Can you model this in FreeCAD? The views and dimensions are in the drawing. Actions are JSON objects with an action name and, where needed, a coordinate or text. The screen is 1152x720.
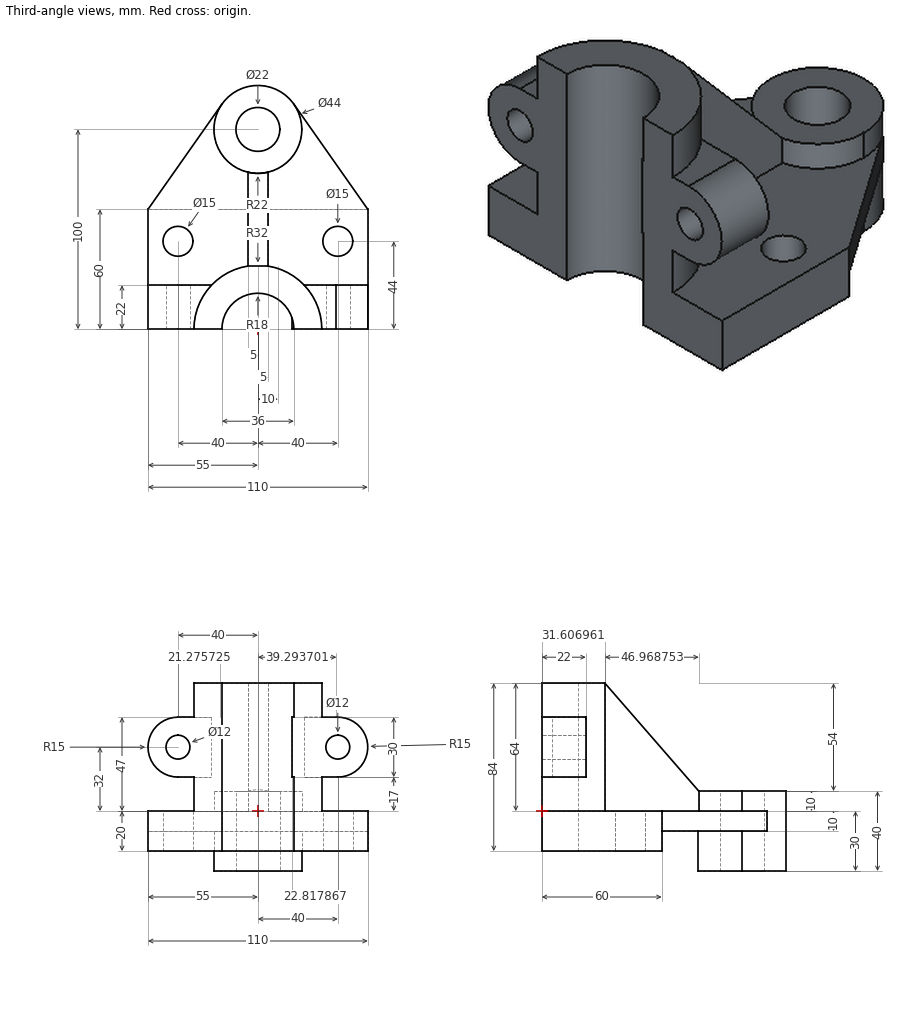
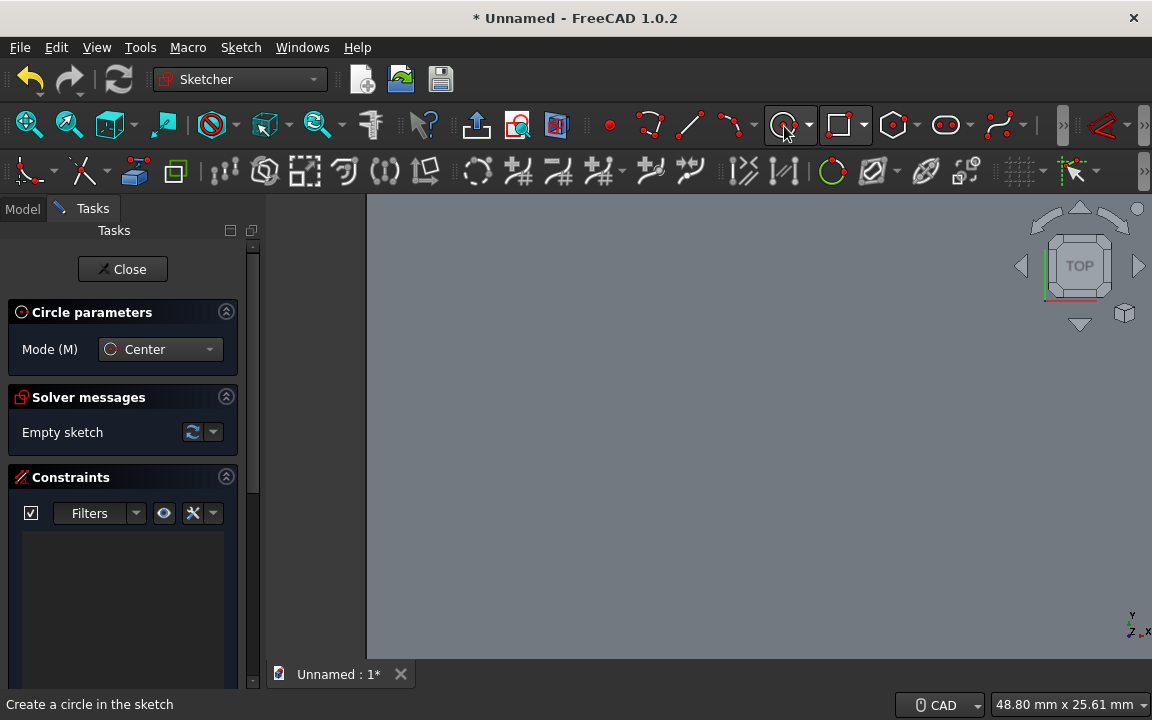
{"action": "left_click", "coordinate": [638, 421]}
{"action": "left_click", "coordinate": [735, 325]}
{"action": "key", "text": "Escape"}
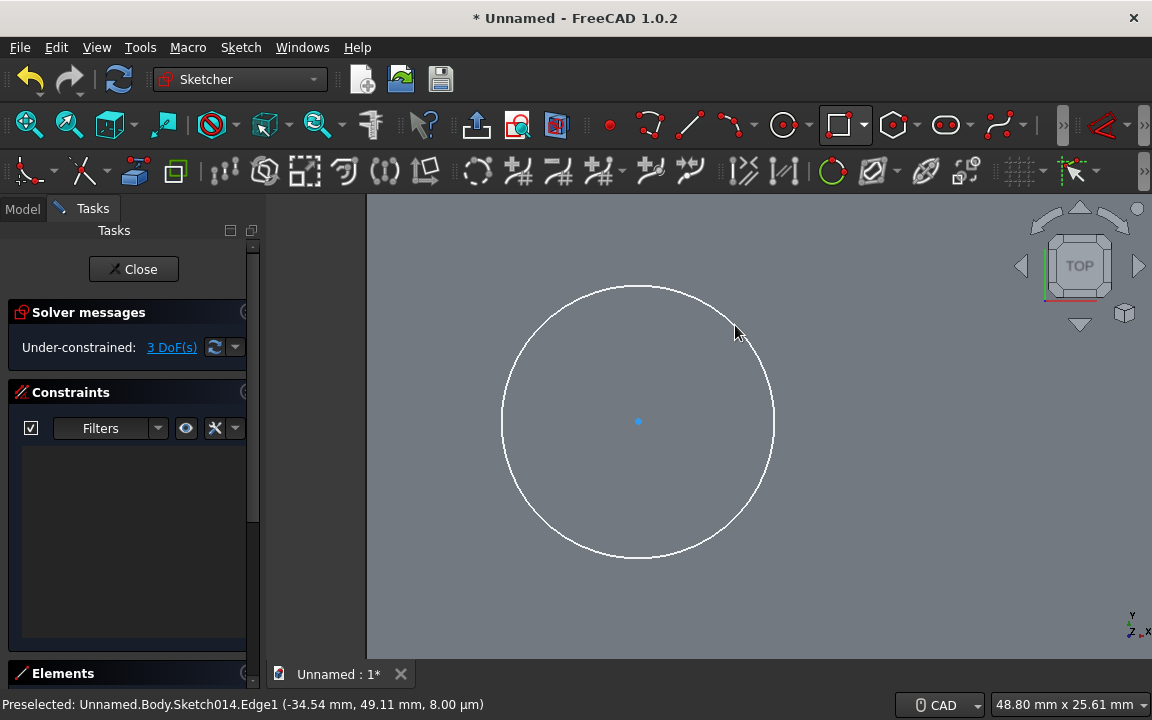
{"action": "left_click", "coordinate": [1102, 126]}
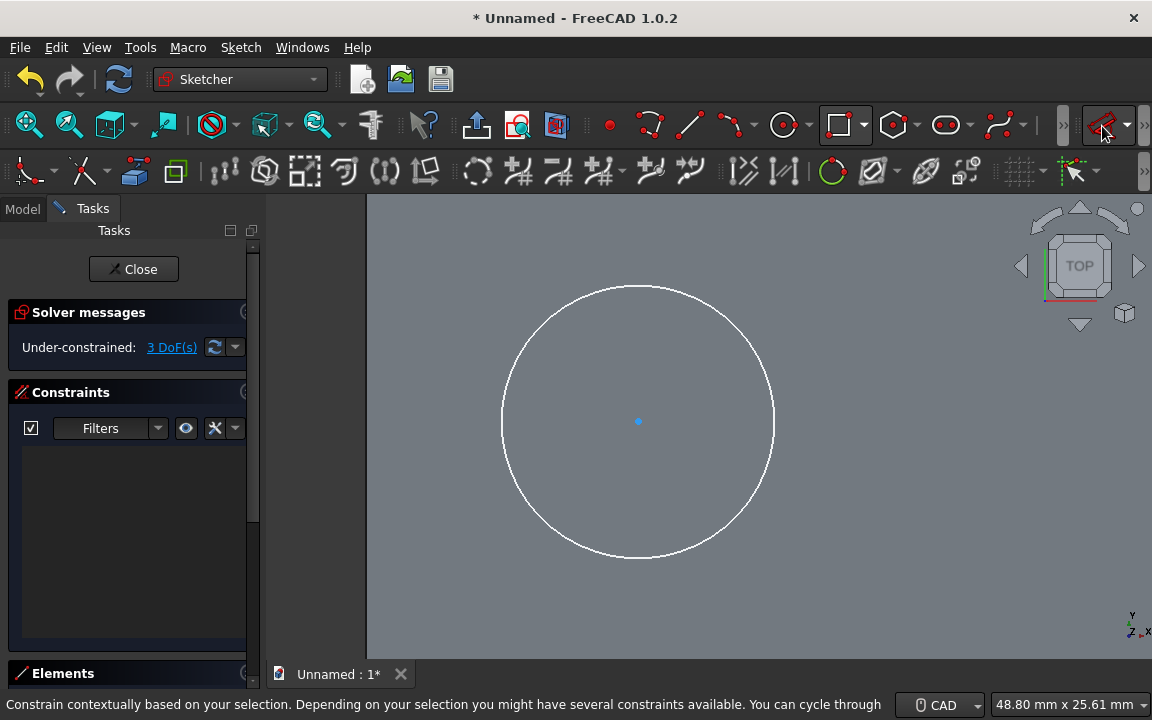
{"action": "left_click", "coordinate": [734, 325]}
{"action": "left_click", "coordinate": [757, 302]}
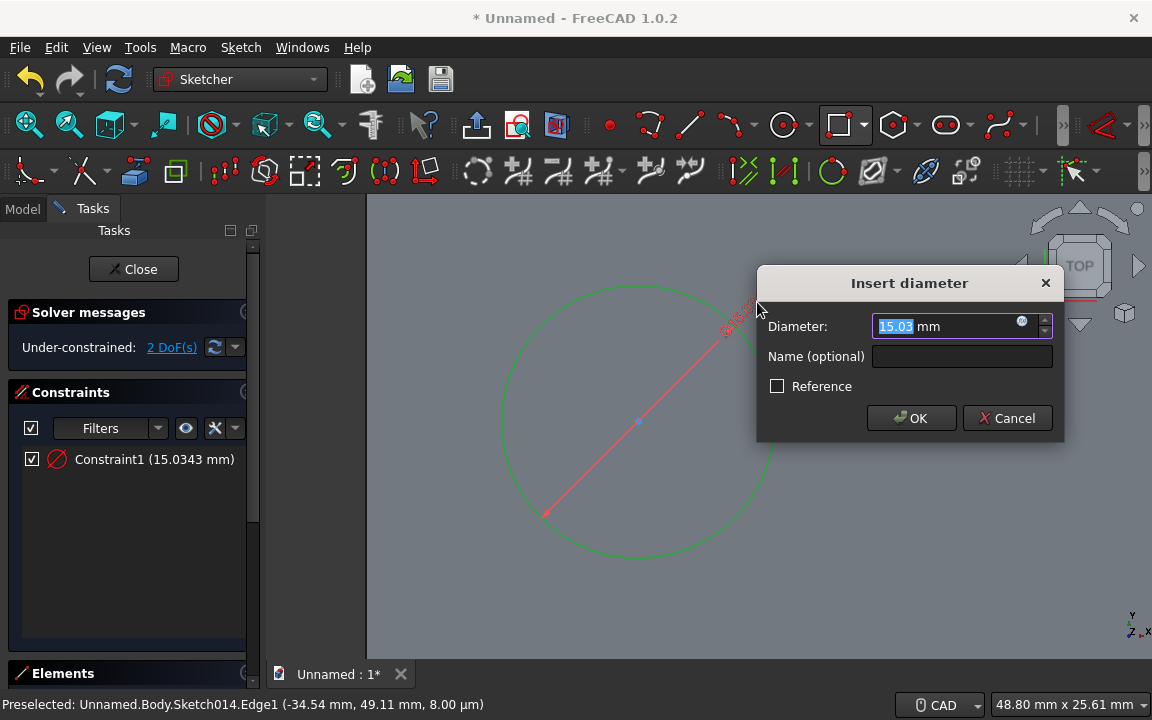
{"action": "type", "text": "15"}
{"action": "key", "text": "Return"}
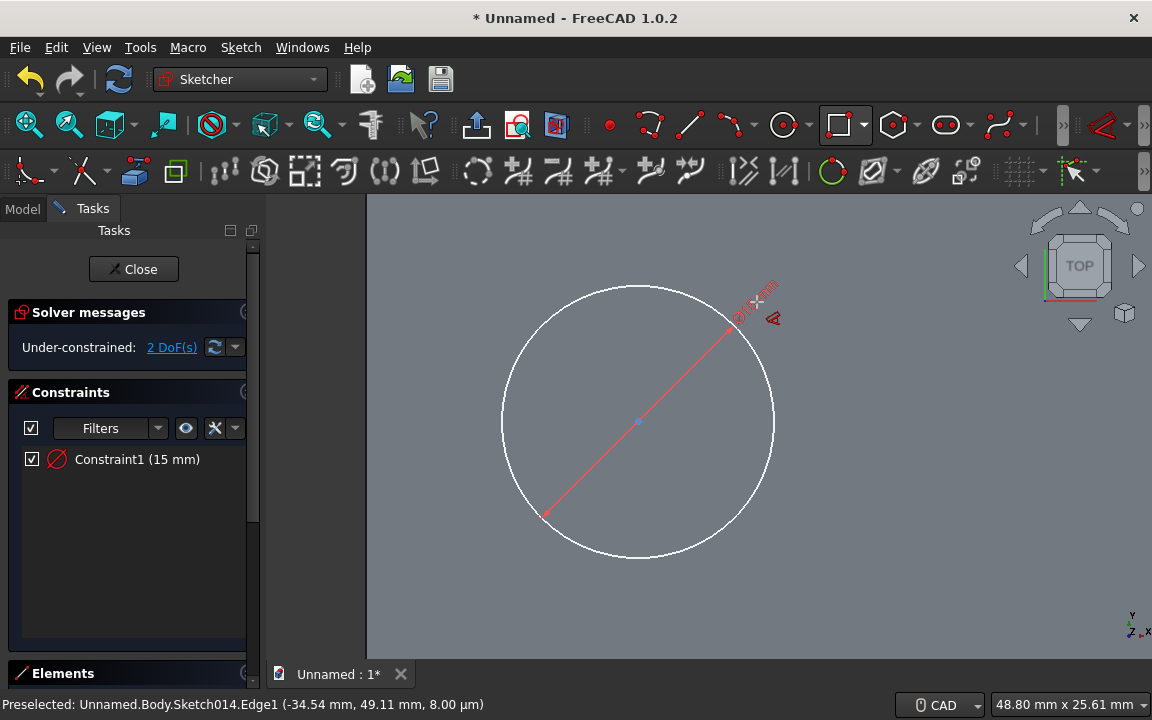
{"action": "left_click", "coordinate": [638, 422]}
{"action": "left_click", "coordinate": [812, 388]}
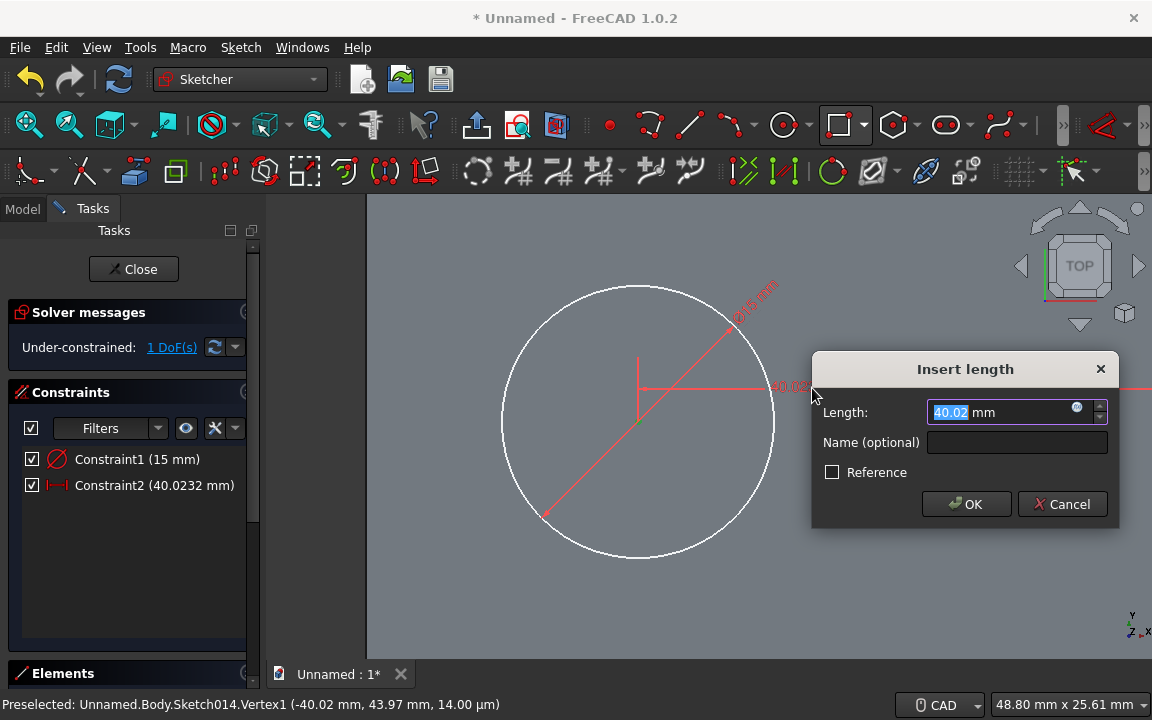
{"action": "type", "text": "40"}
{"action": "key", "text": "Return"}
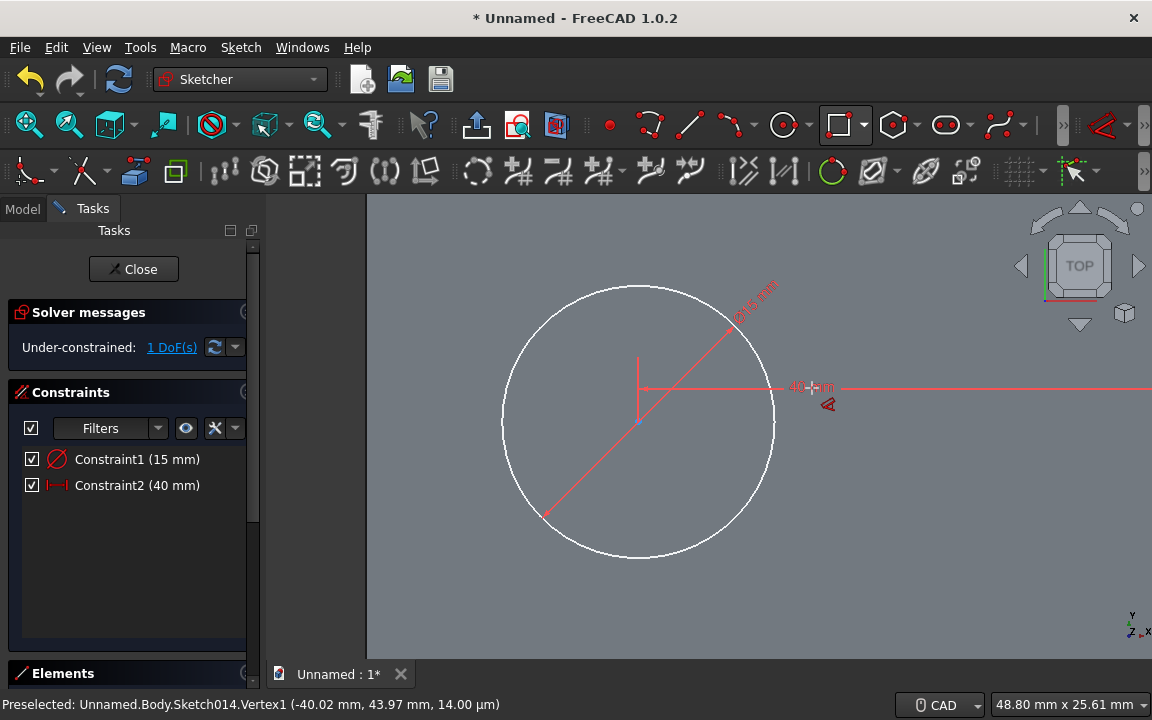
{"action": "left_click", "coordinate": [638, 422]}
{"action": "left_click", "coordinate": [604, 526]}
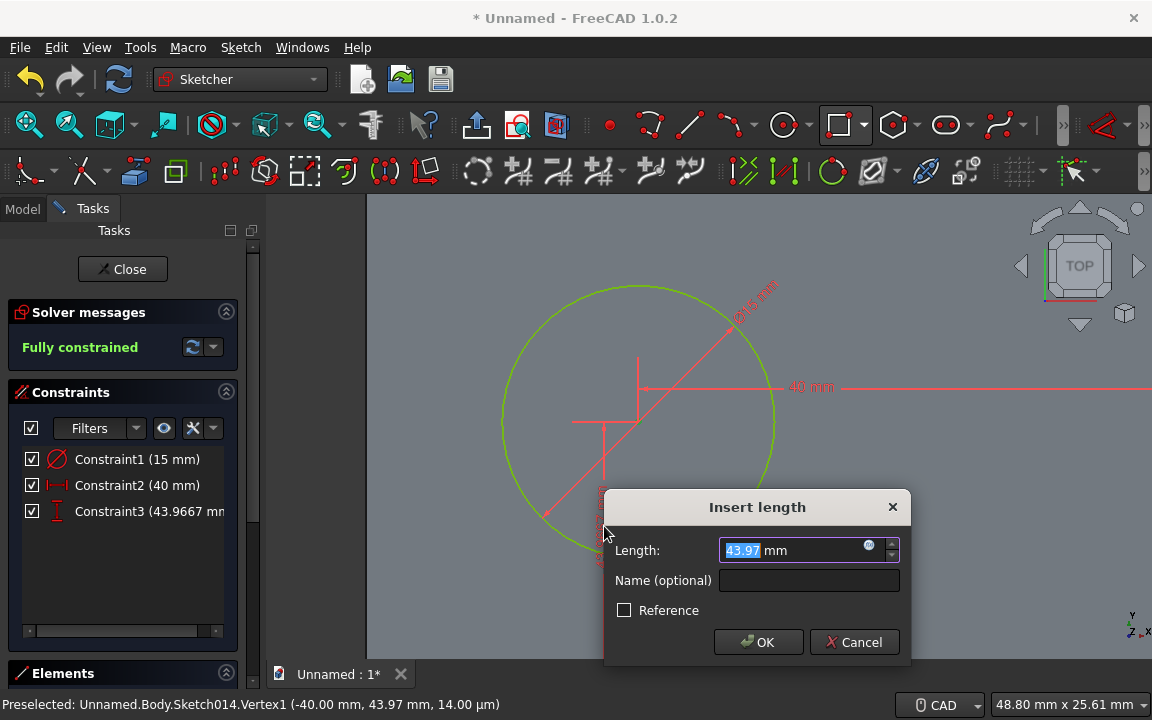
{"action": "type", "text": "44"}
{"action": "key", "text": "Return"}
{"action": "key", "text": "Escape"}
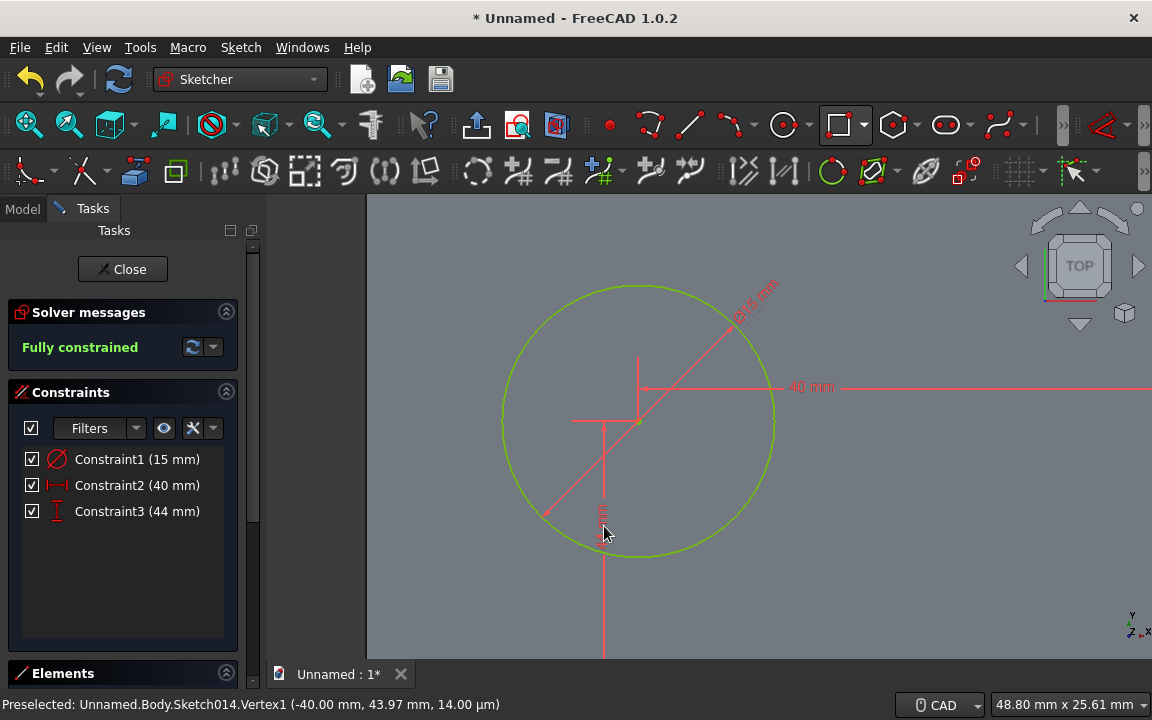
{"action": "left_click", "coordinate": [123, 269]}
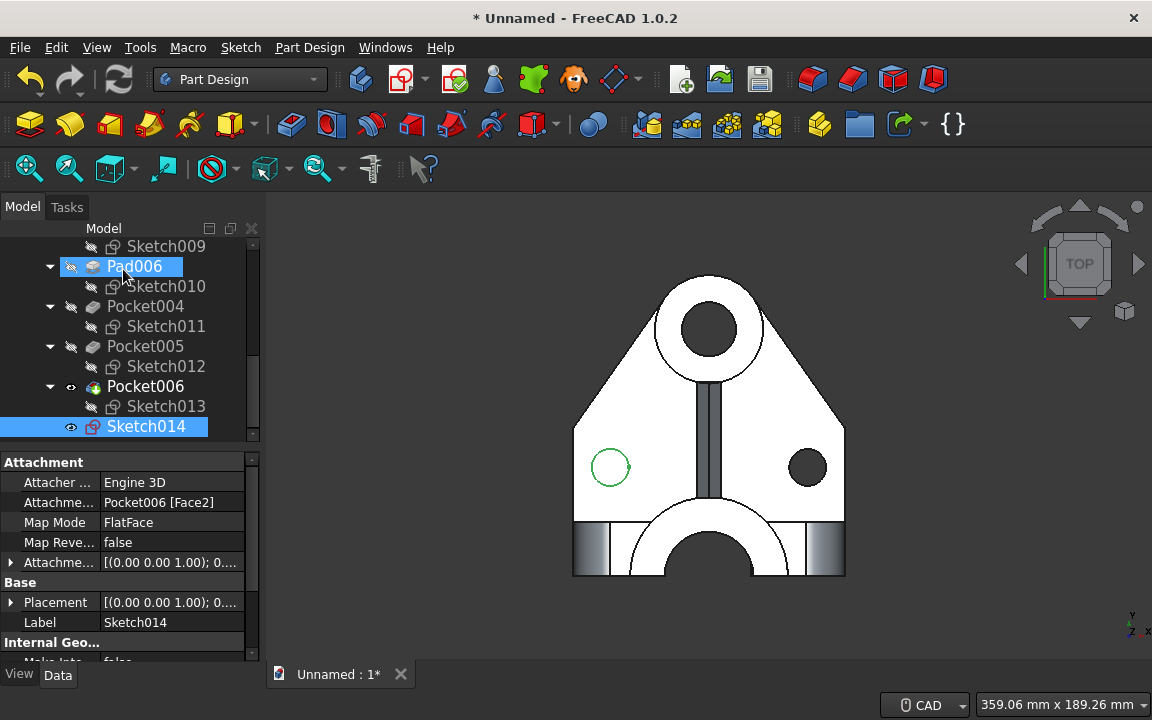
{"action": "left_click", "coordinate": [292, 124]}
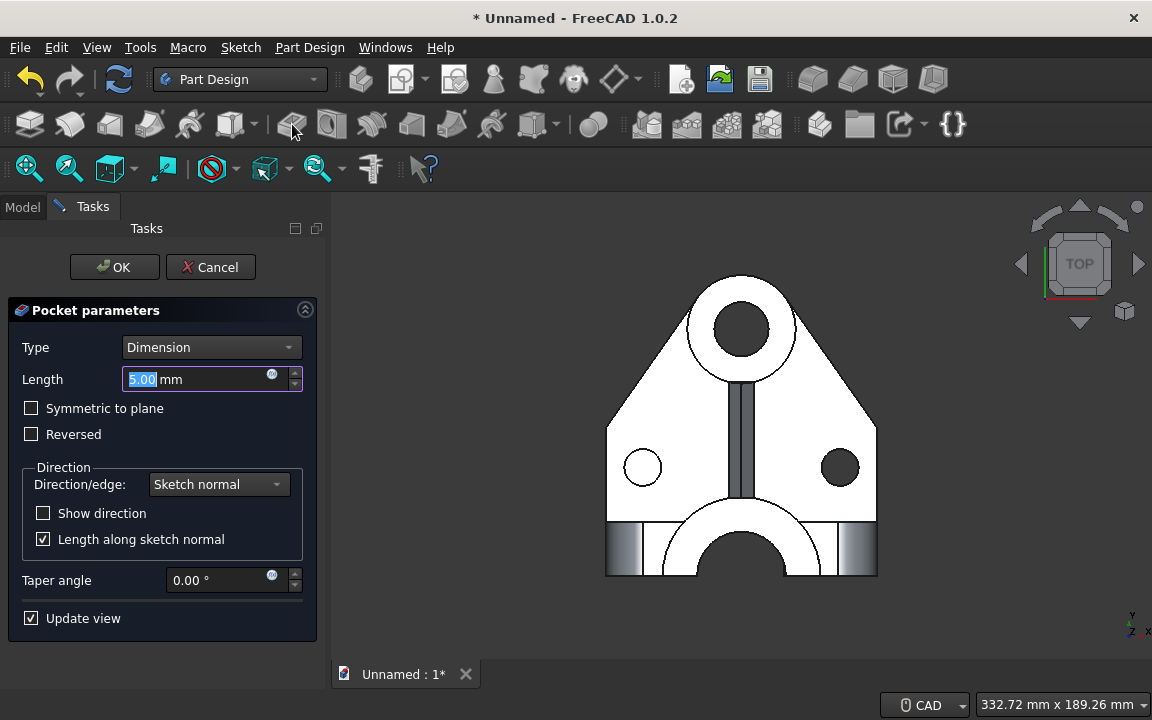
{"action": "type", "text": "20"}
{"action": "key", "text": "Tab"}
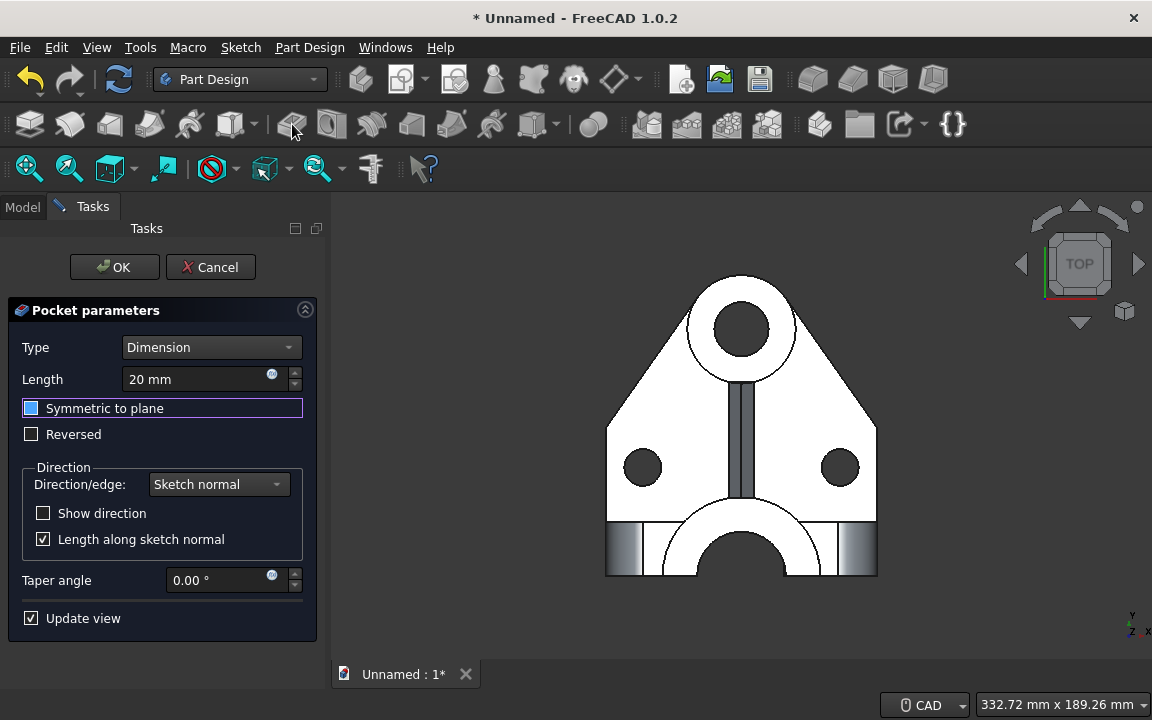
{"action": "left_click", "coordinate": [115, 267]}